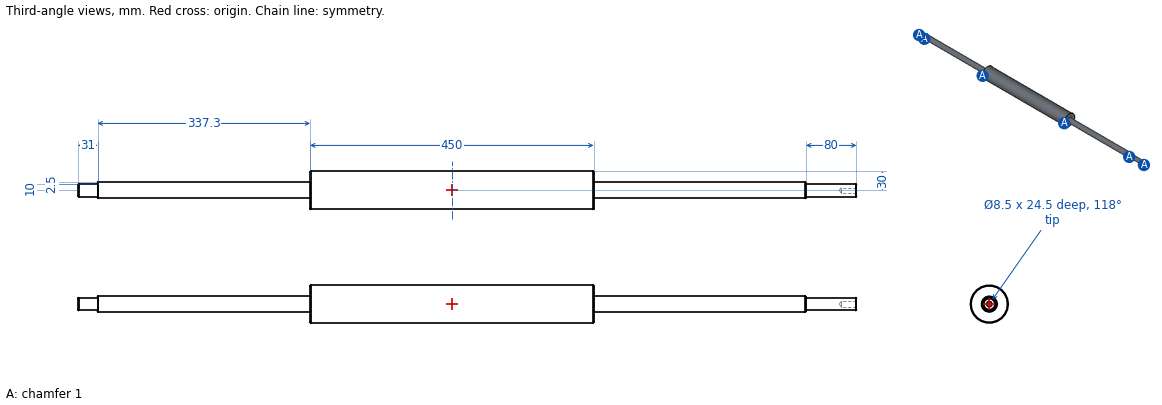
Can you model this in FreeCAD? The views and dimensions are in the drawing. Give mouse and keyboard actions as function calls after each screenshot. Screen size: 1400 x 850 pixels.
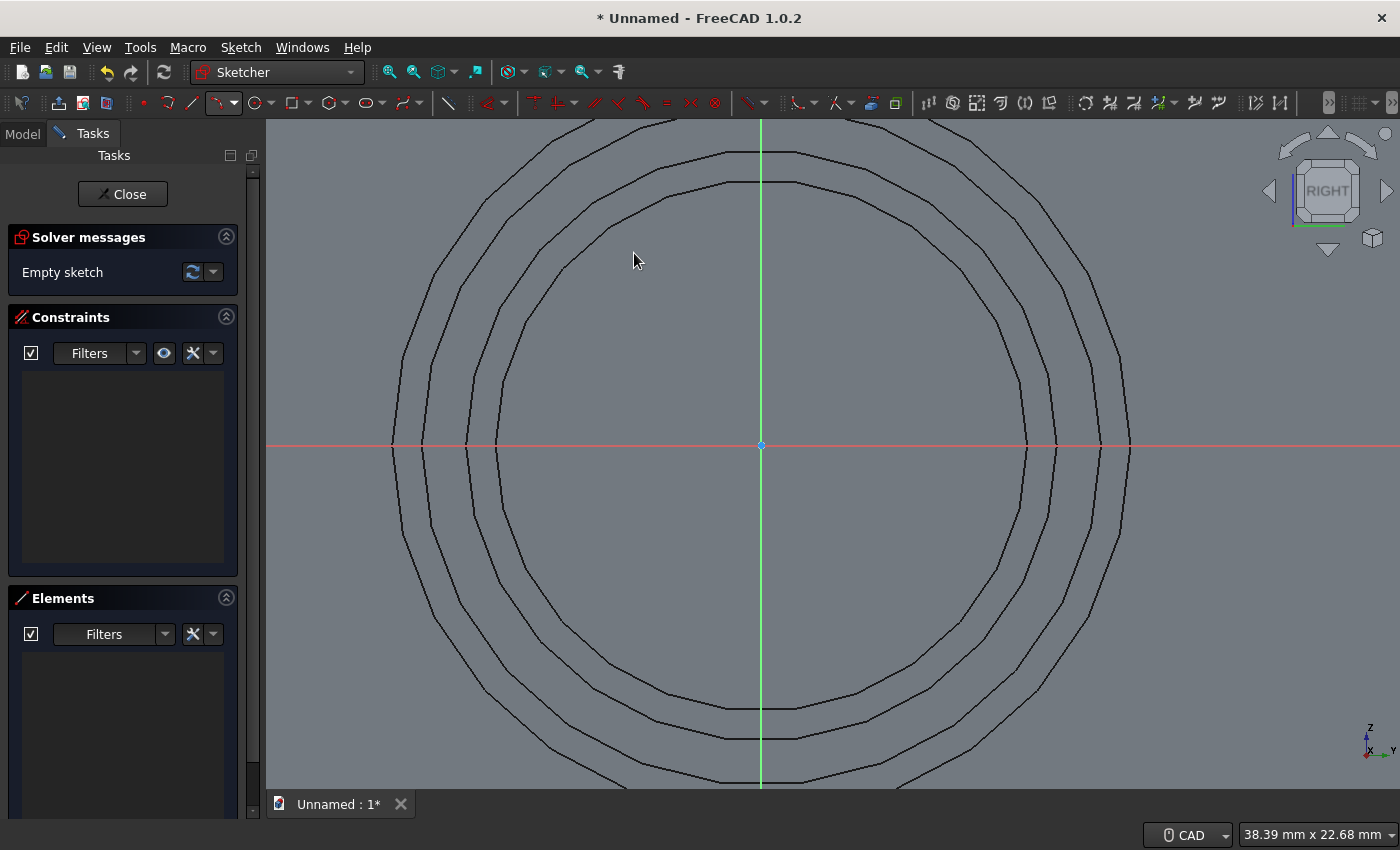
scroll(758, 435, up, 3)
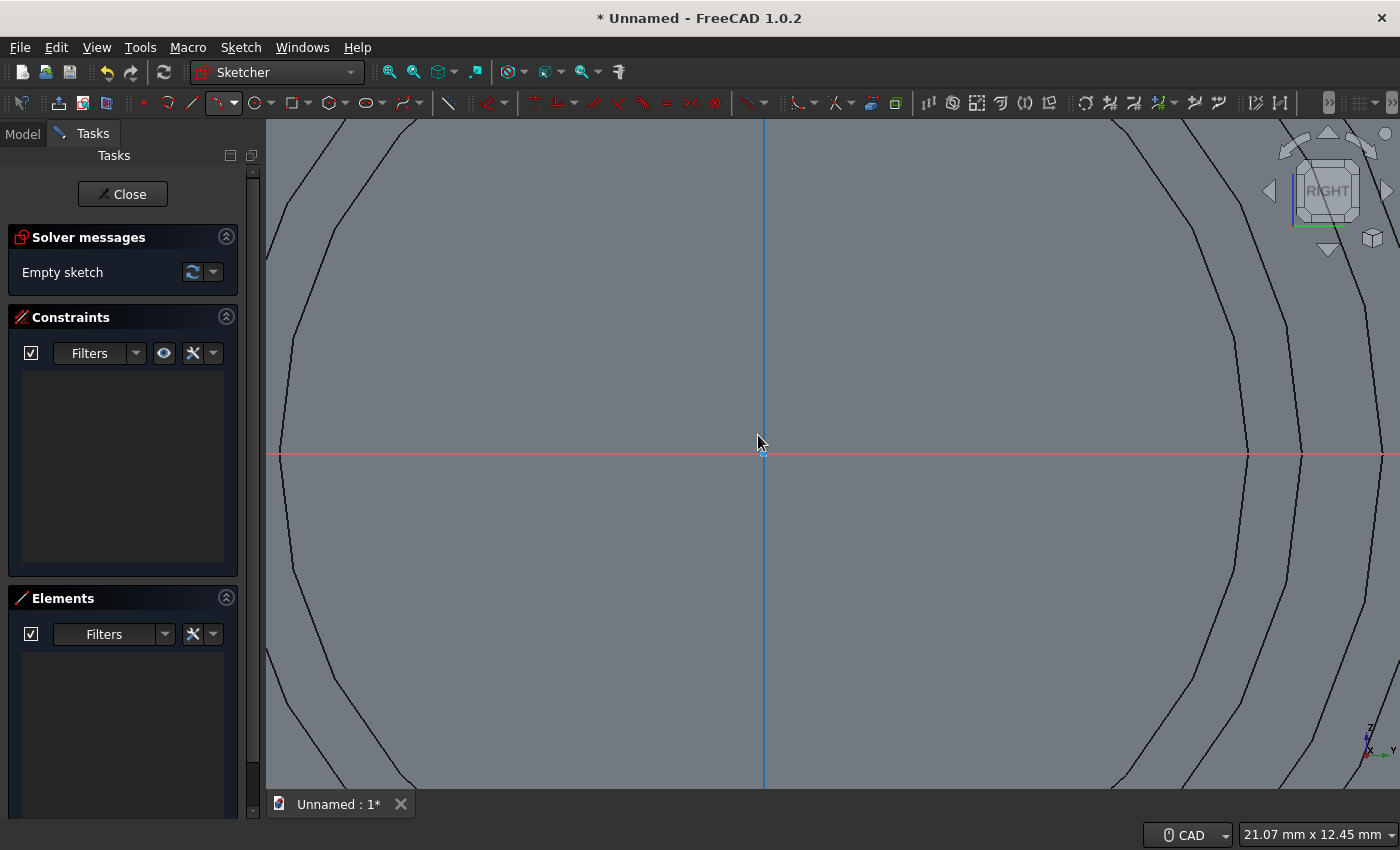
click(256, 104)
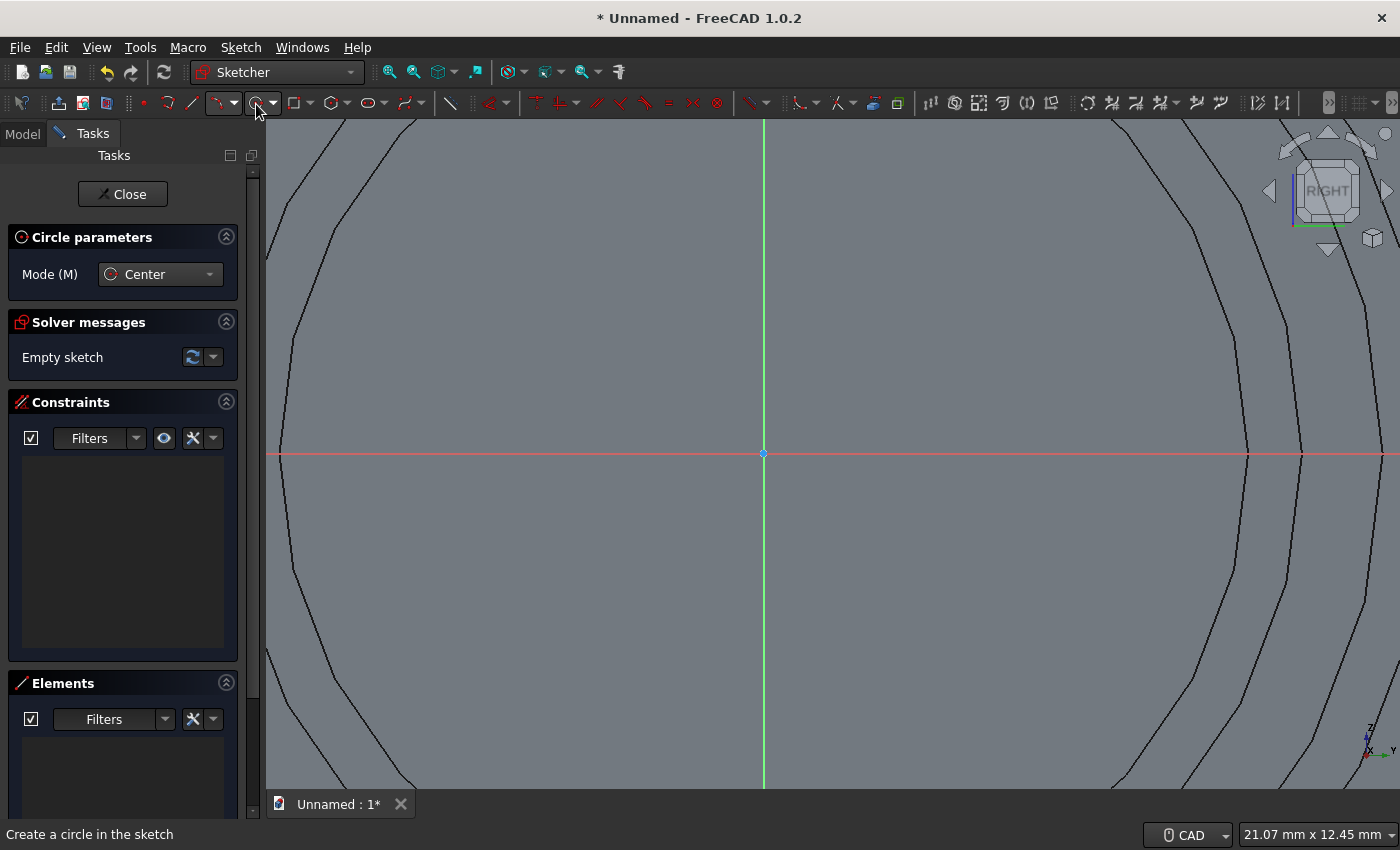
click(764, 454)
click(926, 292)
key(Escape)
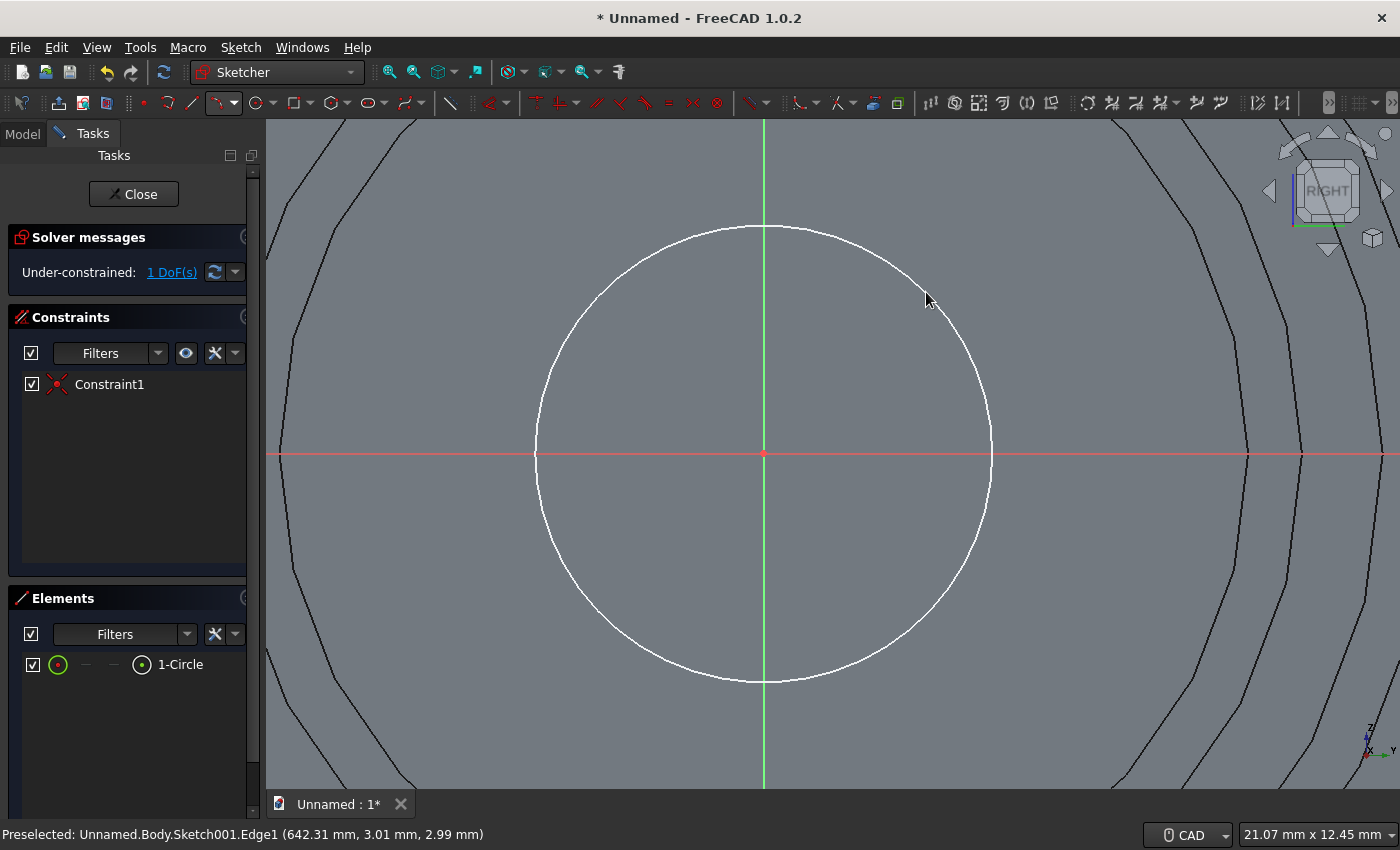
key(d)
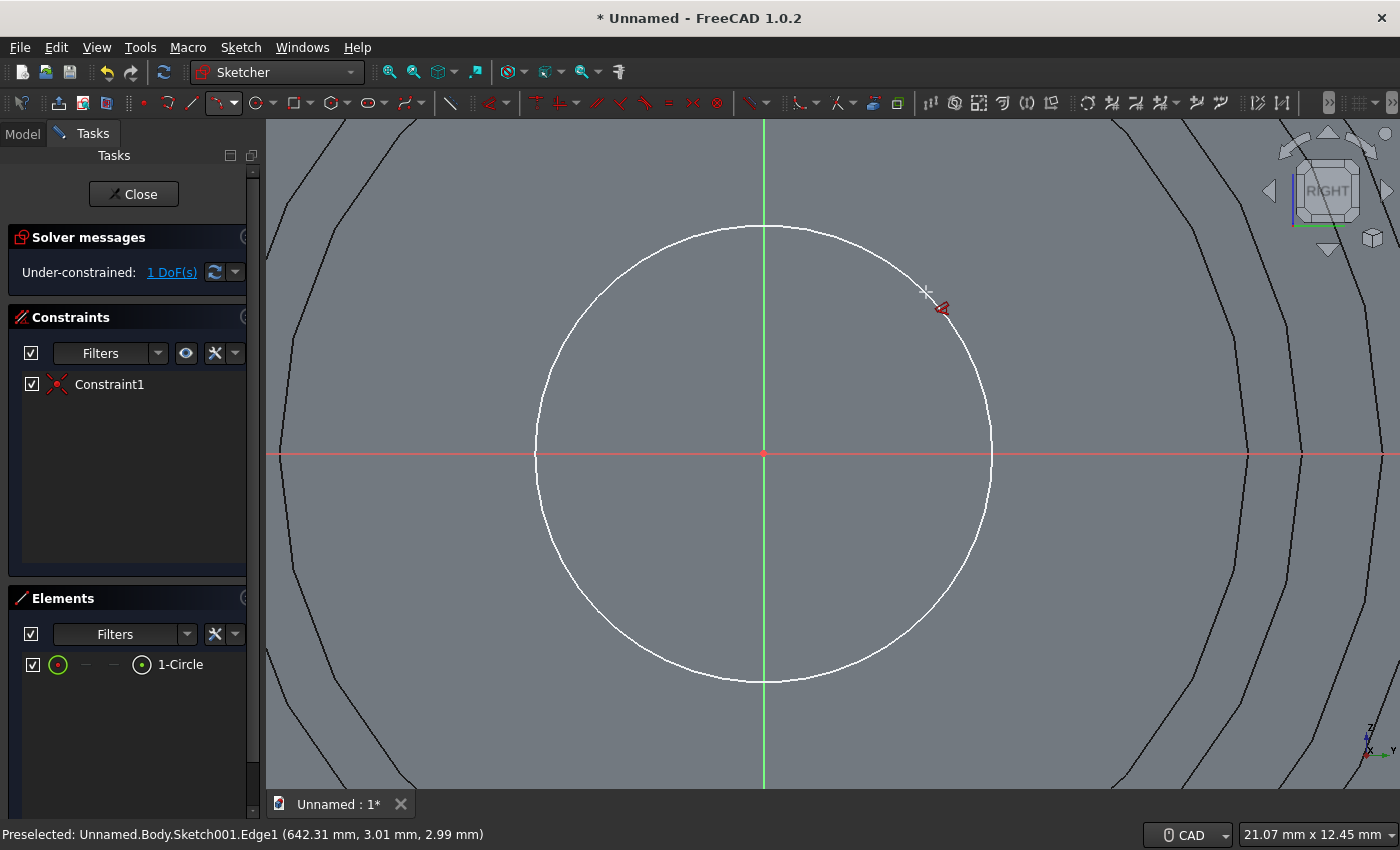
click(925, 292)
click(948, 269)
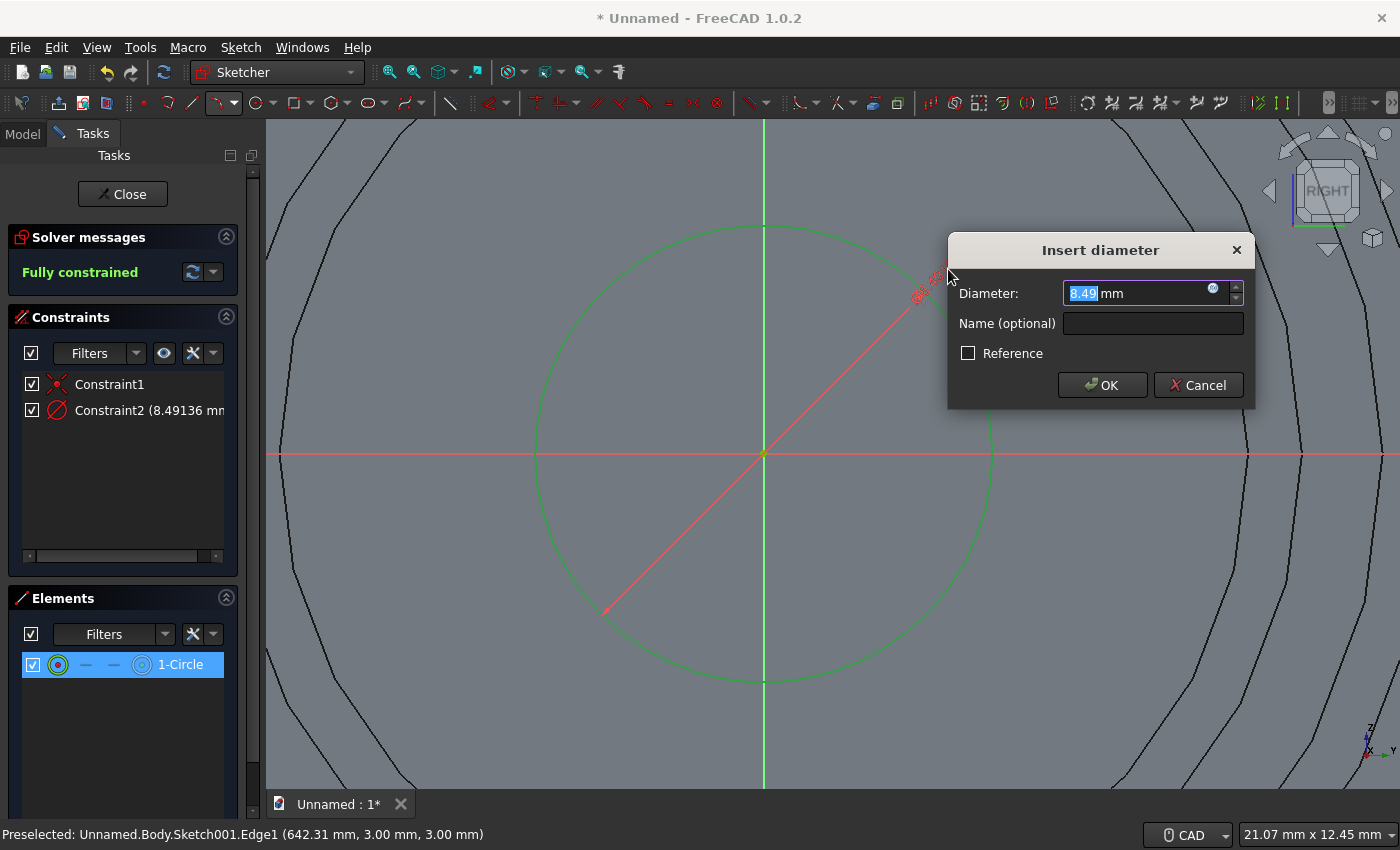
text(8.5)
key(Return)
key(Escape)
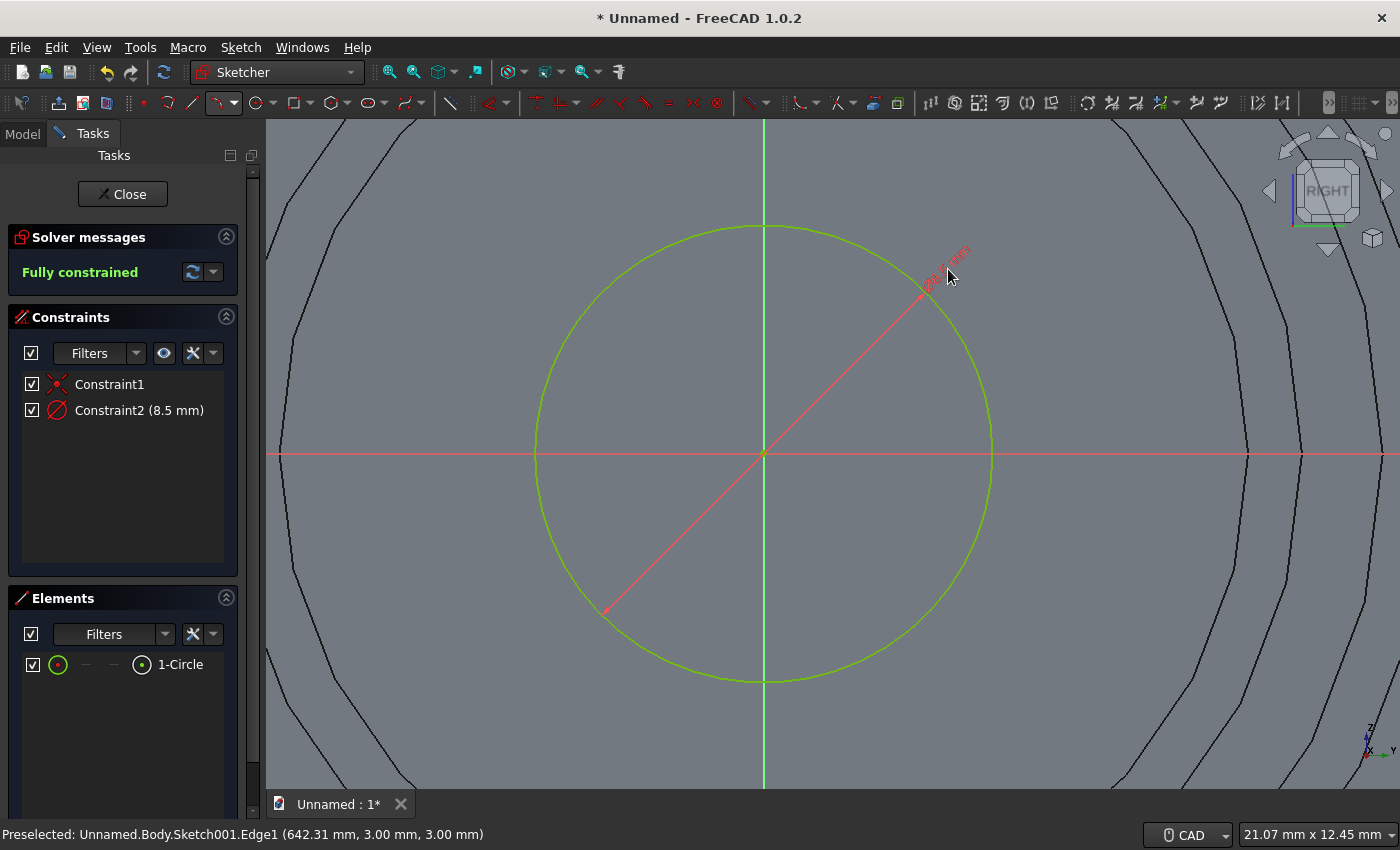
click(123, 194)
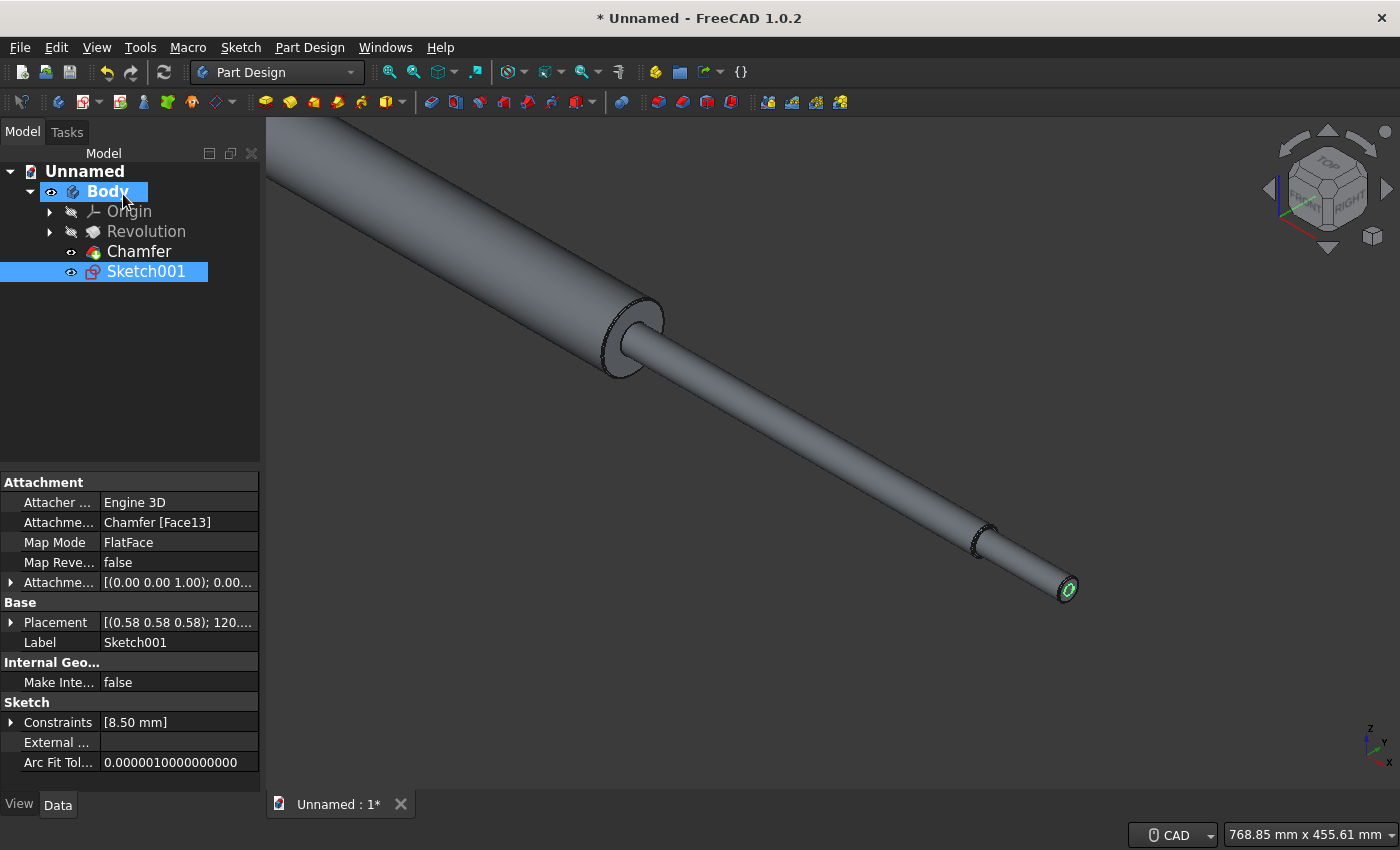
click(456, 102)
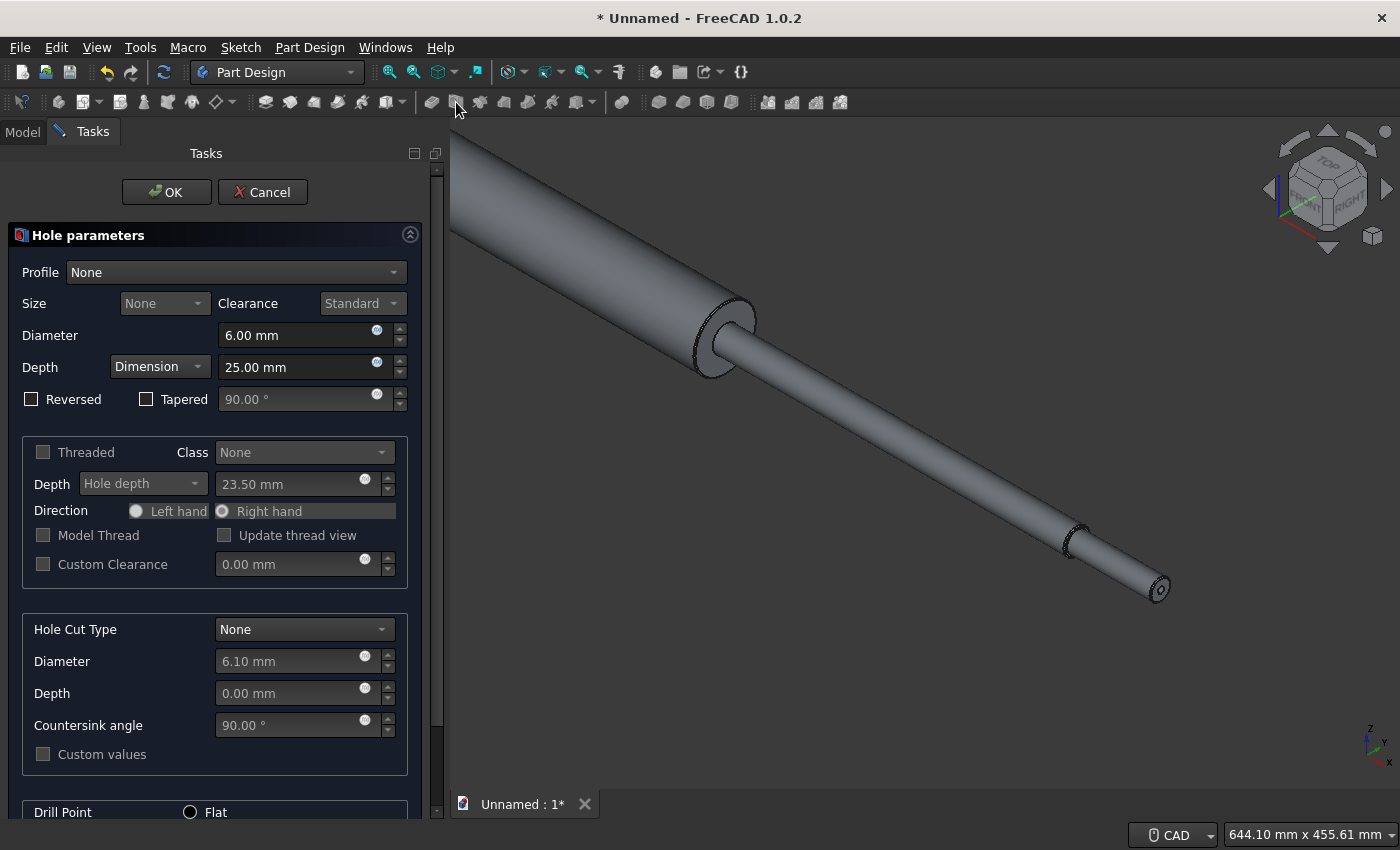
triple_click(305, 335)